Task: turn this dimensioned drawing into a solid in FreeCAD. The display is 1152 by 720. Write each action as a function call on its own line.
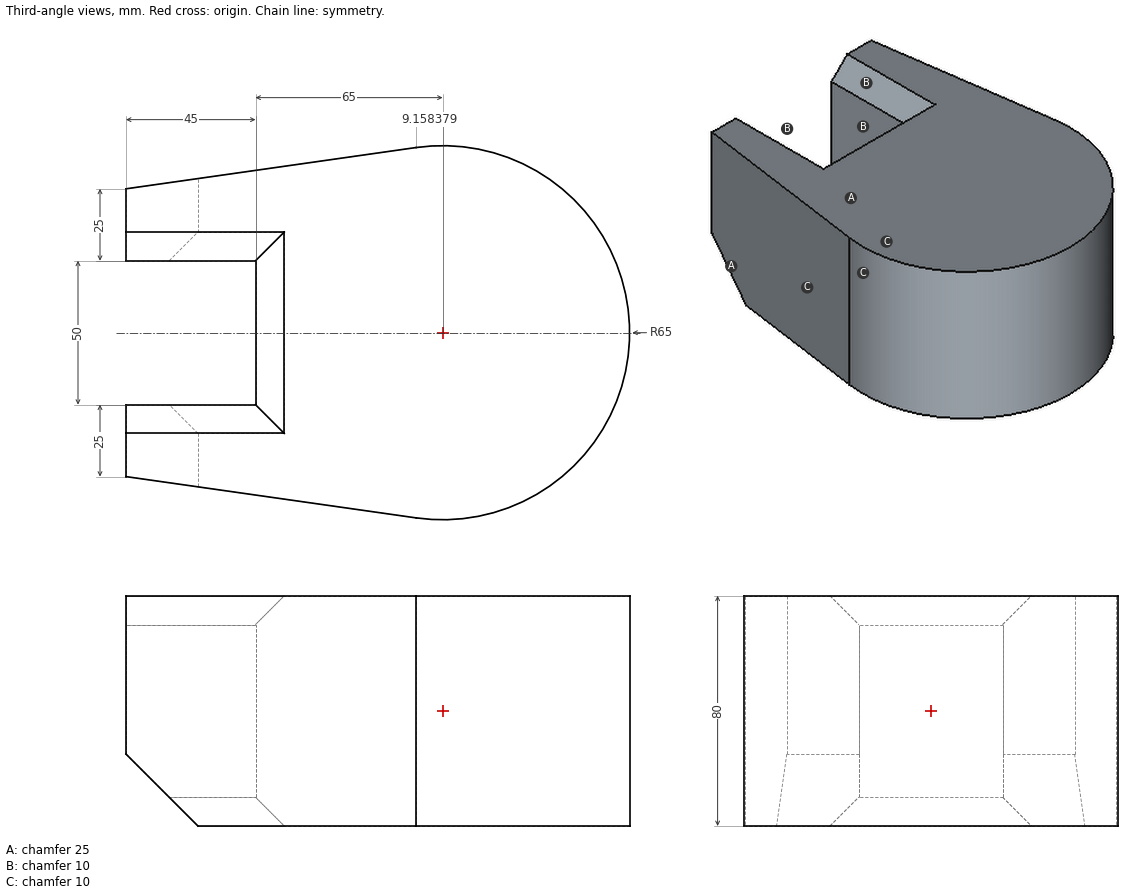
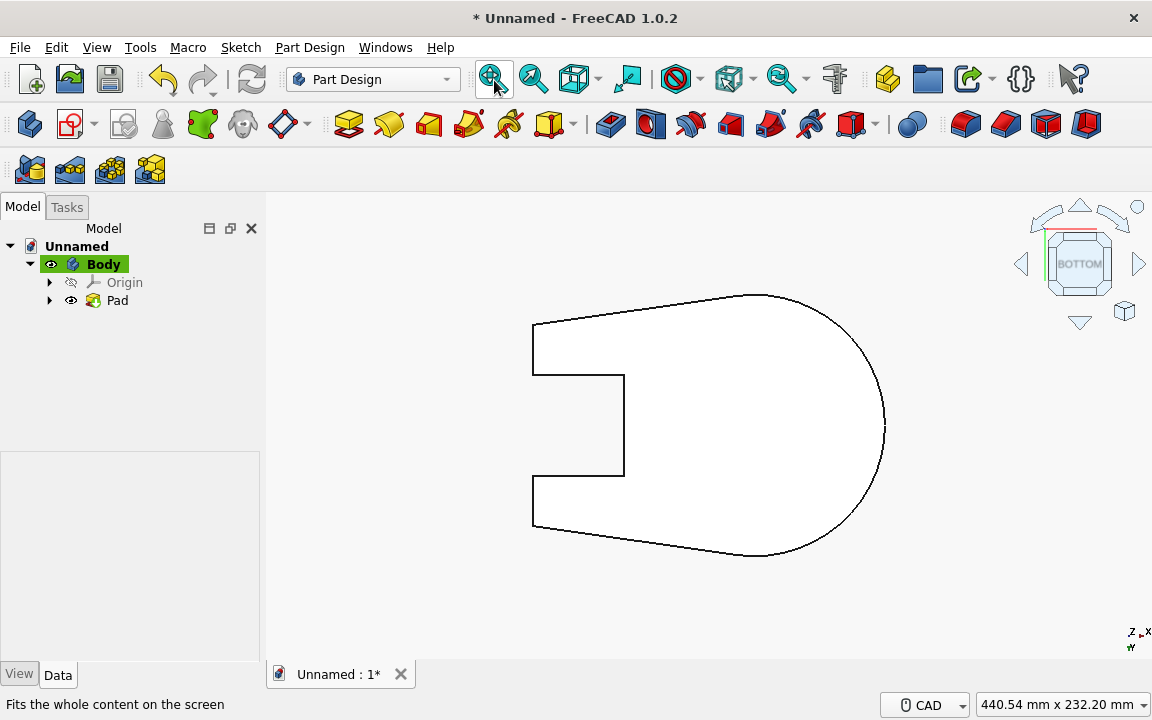
click(533, 500)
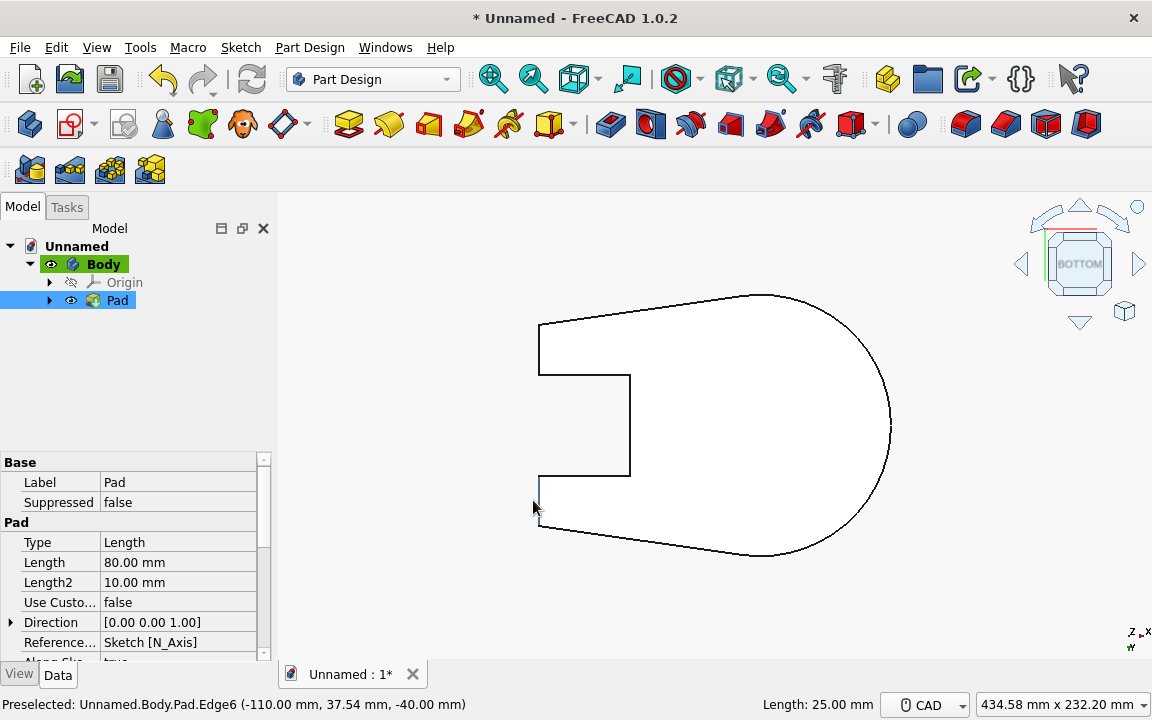
click(539, 349, ctrl)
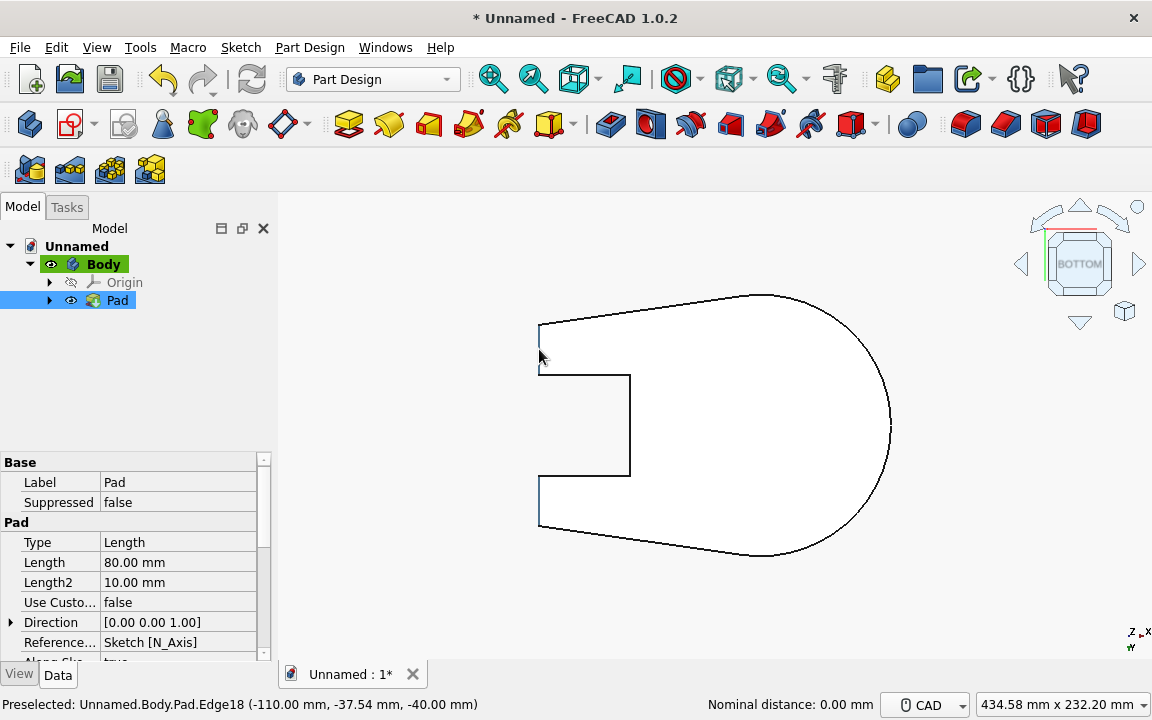
click(1006, 124)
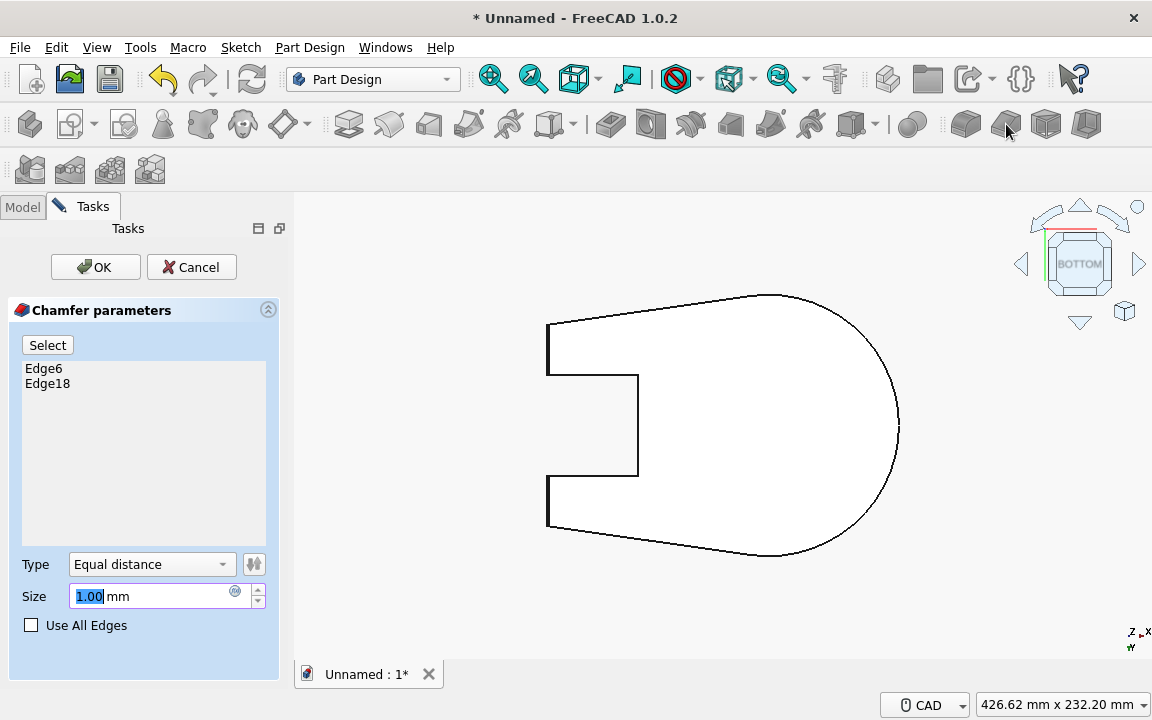
text(25)
key(Tab)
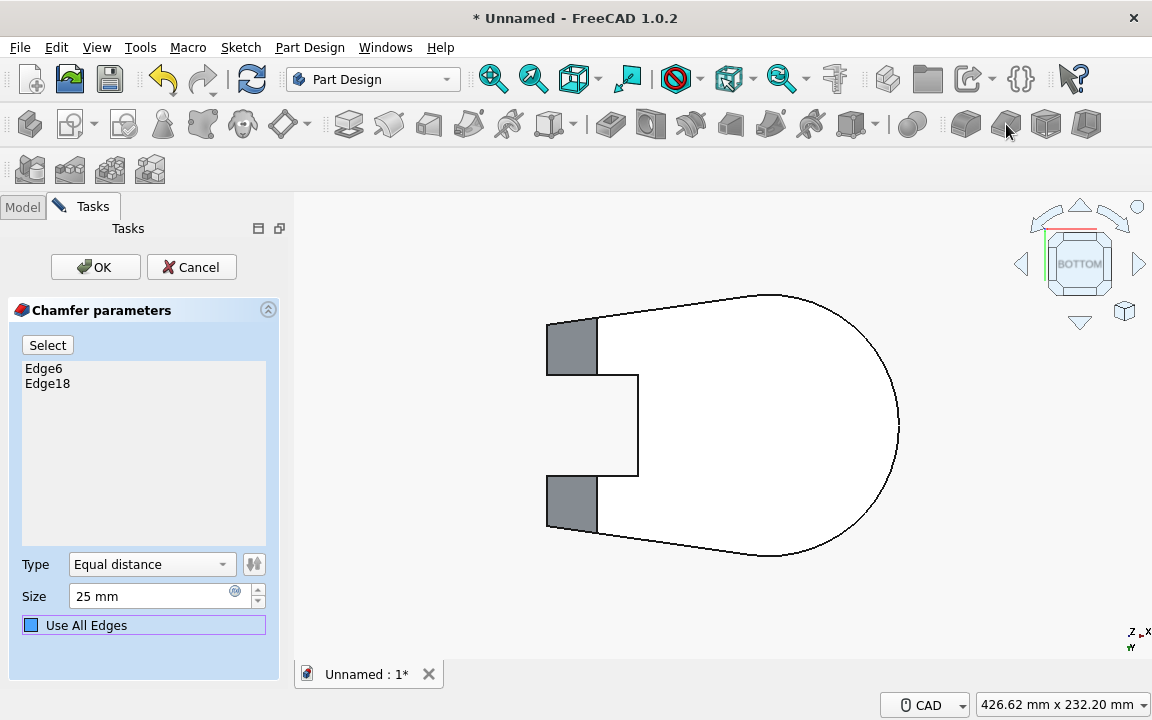
click(96, 267)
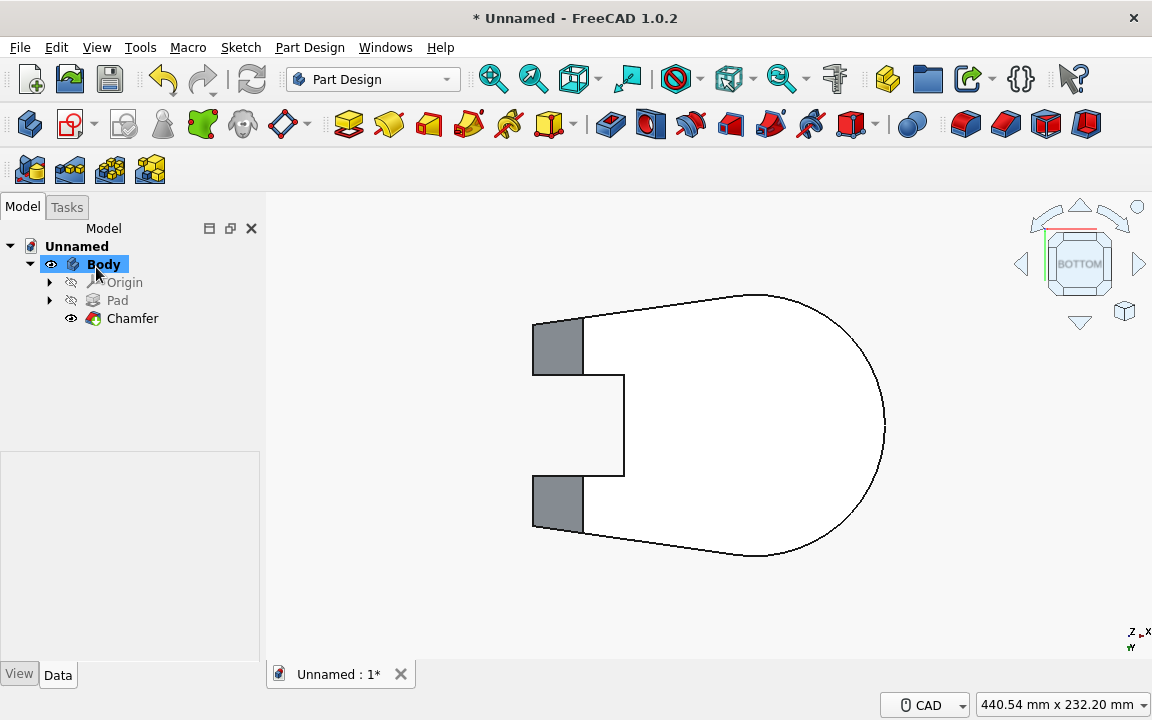
key(0)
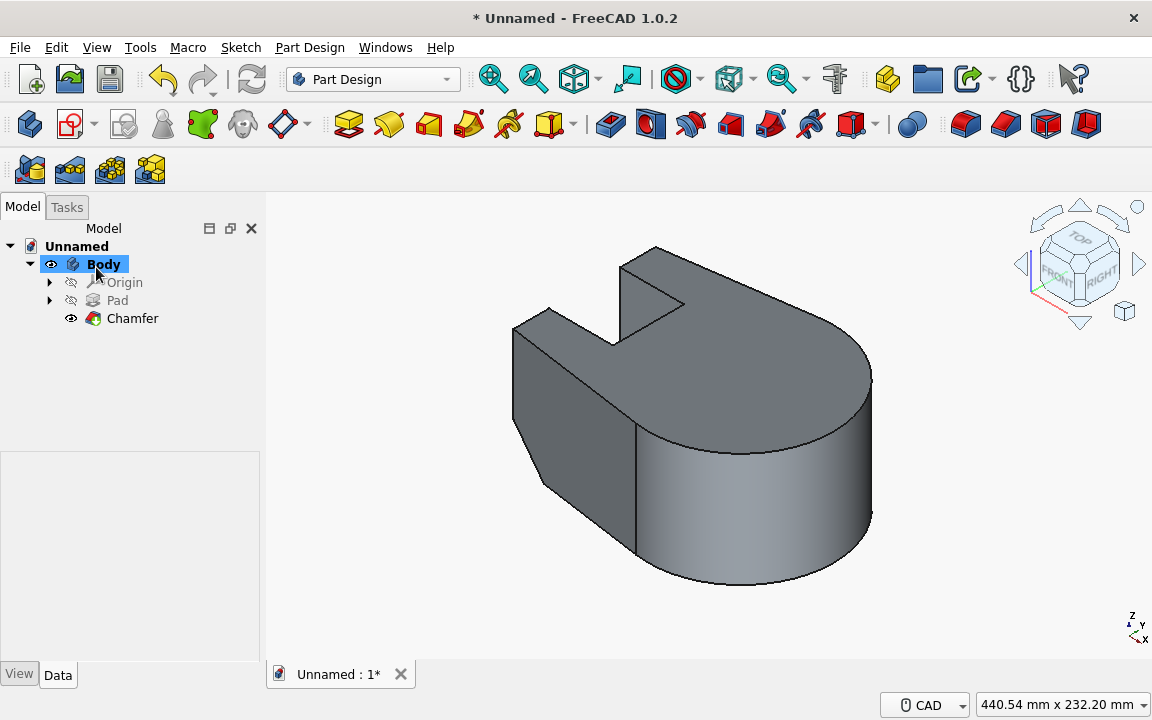
click(652, 285)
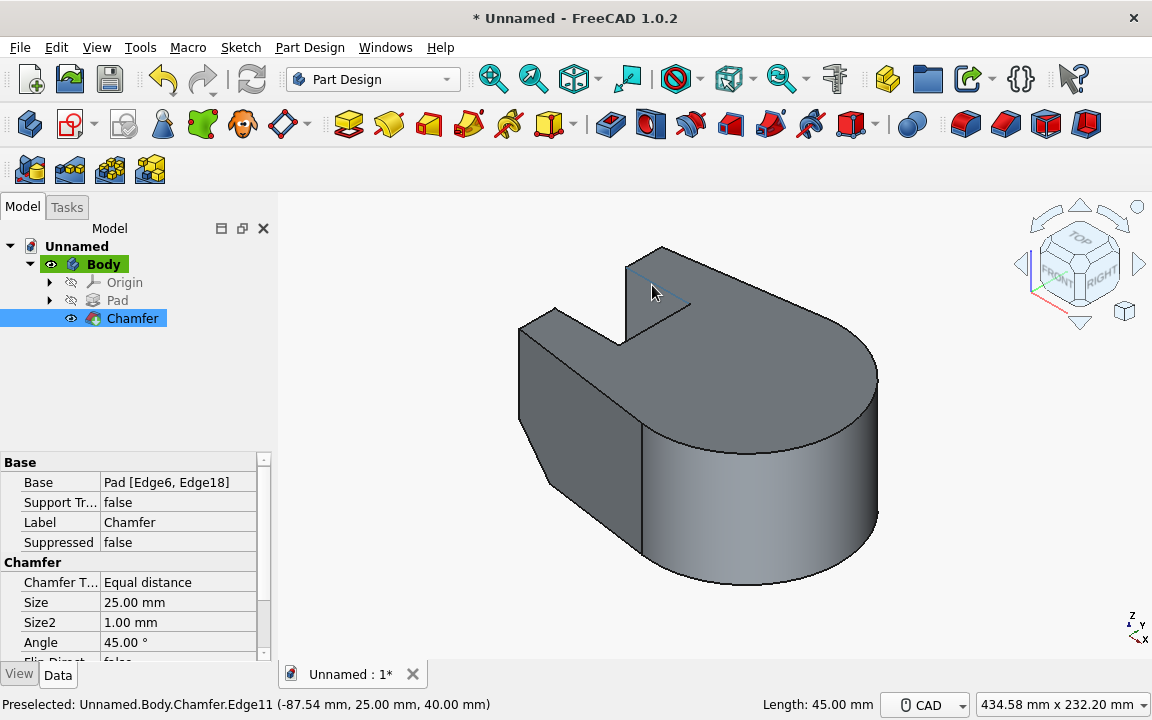
key(2)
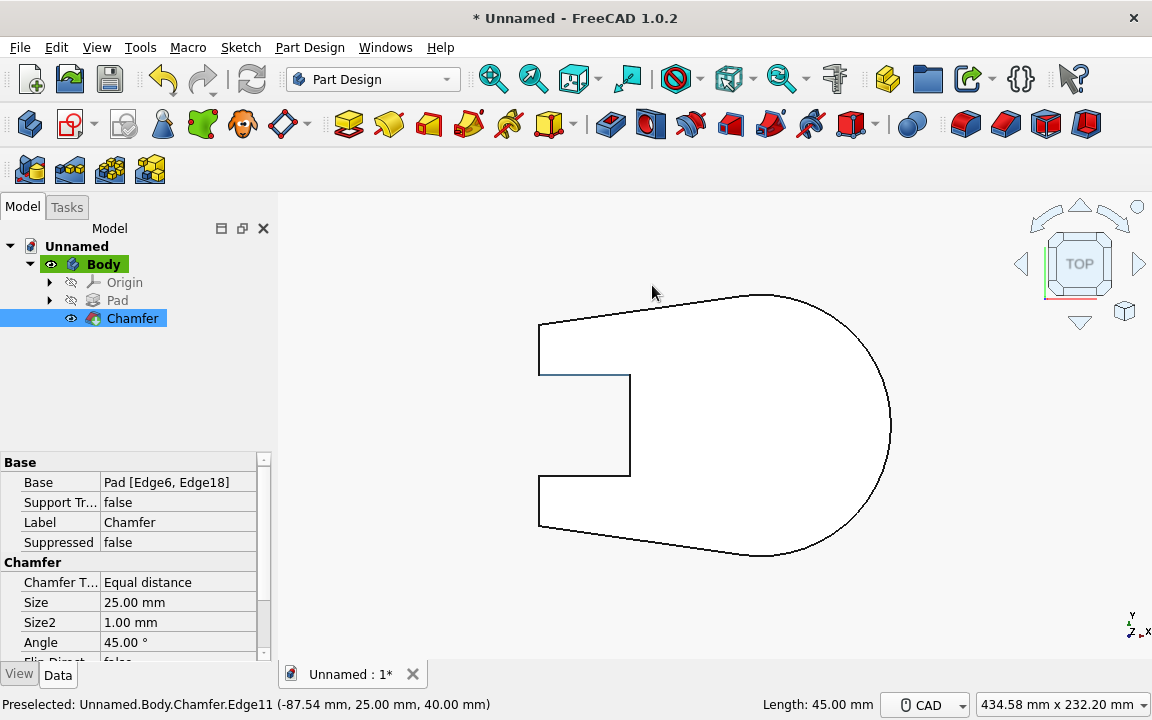
click(630, 425, ctrl)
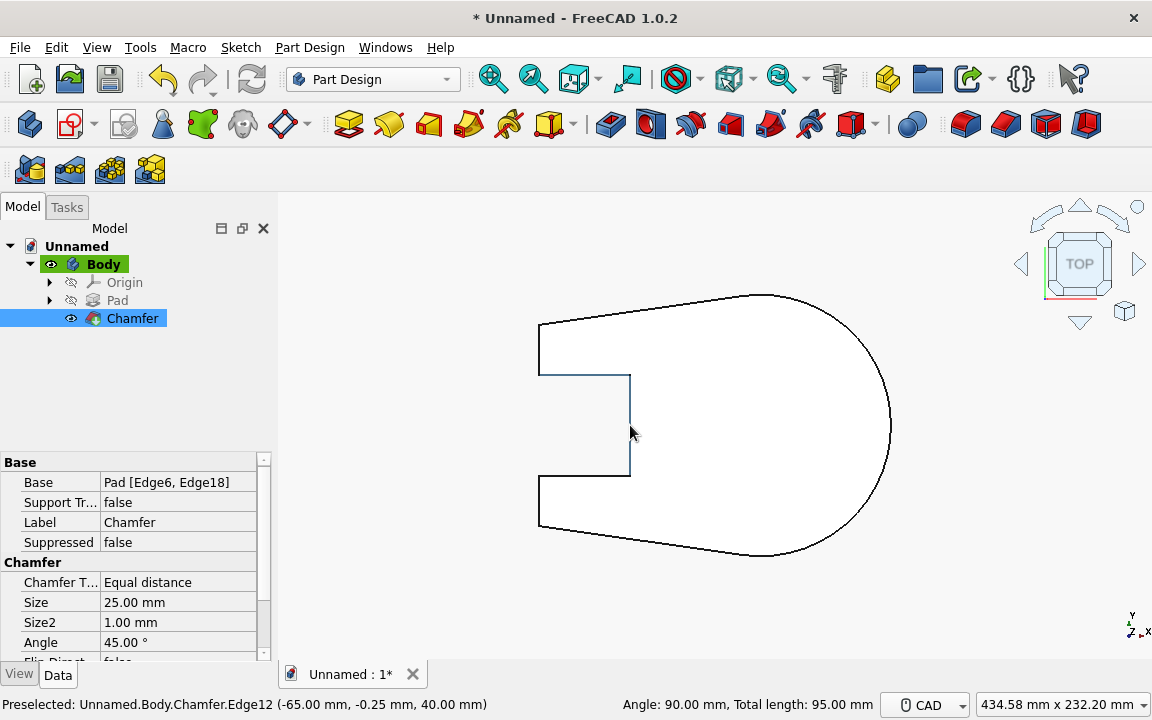
click(584, 475, ctrl)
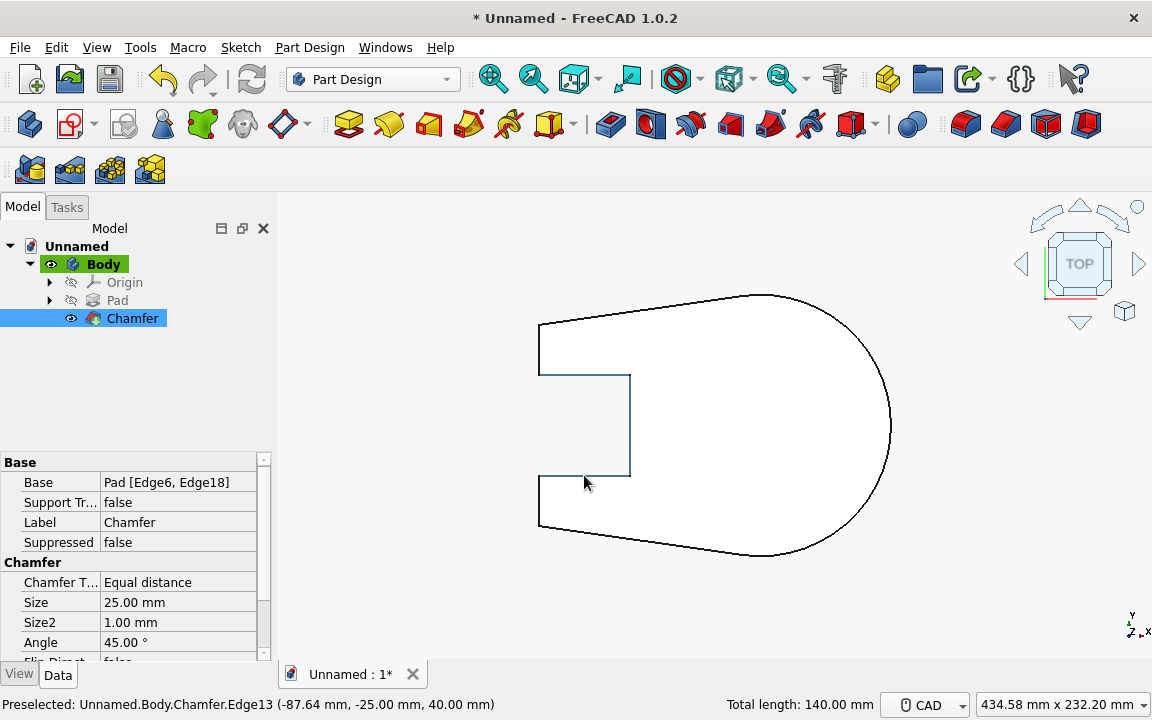
click(1006, 124)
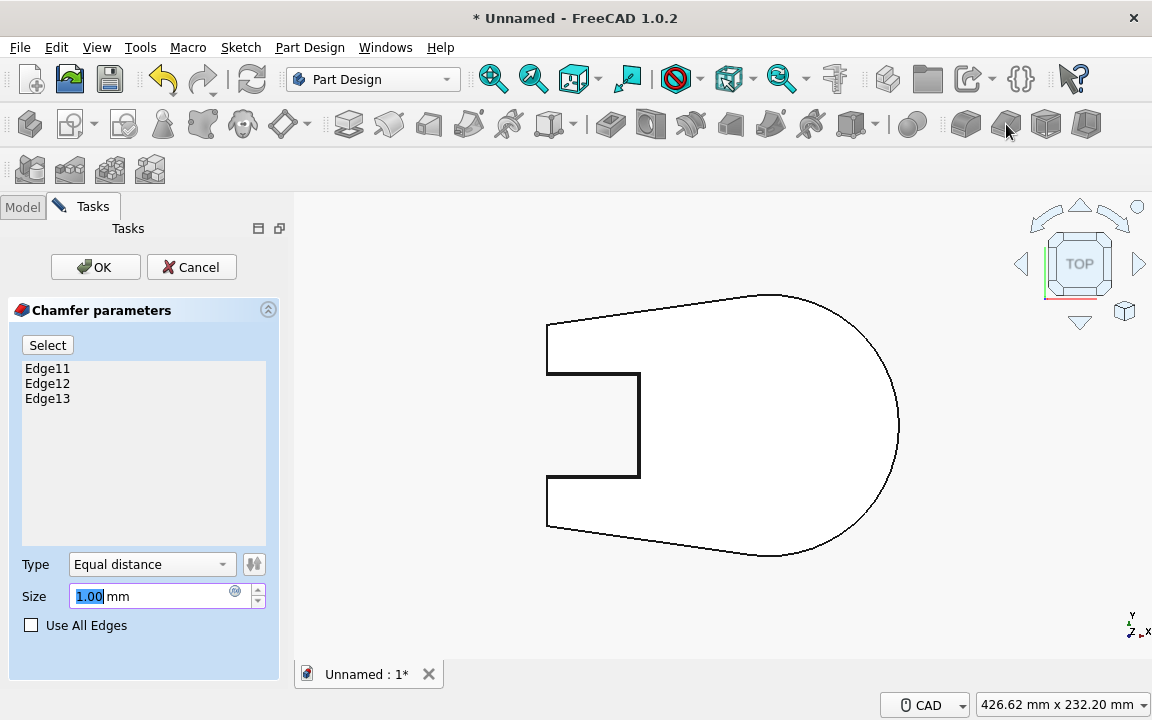
text(10)
key(Tab)